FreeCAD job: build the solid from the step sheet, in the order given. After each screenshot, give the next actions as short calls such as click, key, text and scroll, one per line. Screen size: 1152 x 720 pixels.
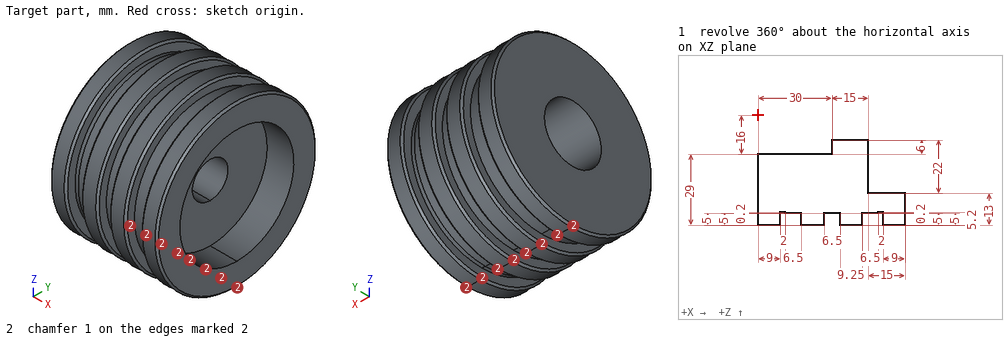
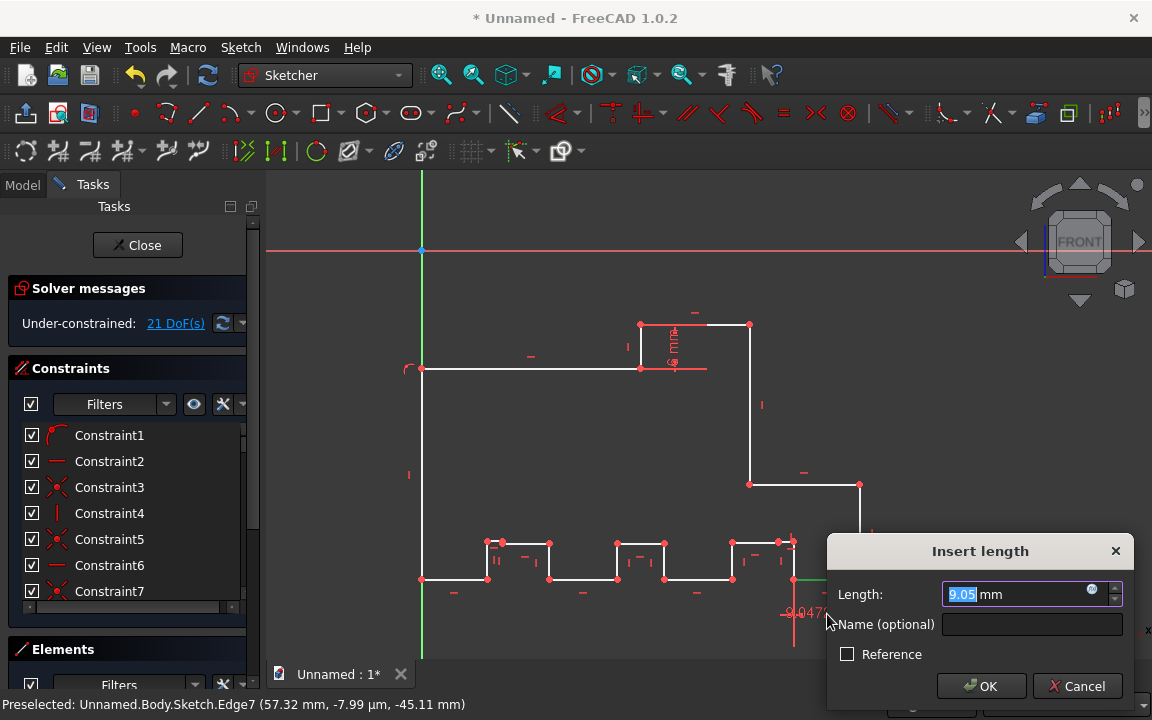
text(9)
key(Return)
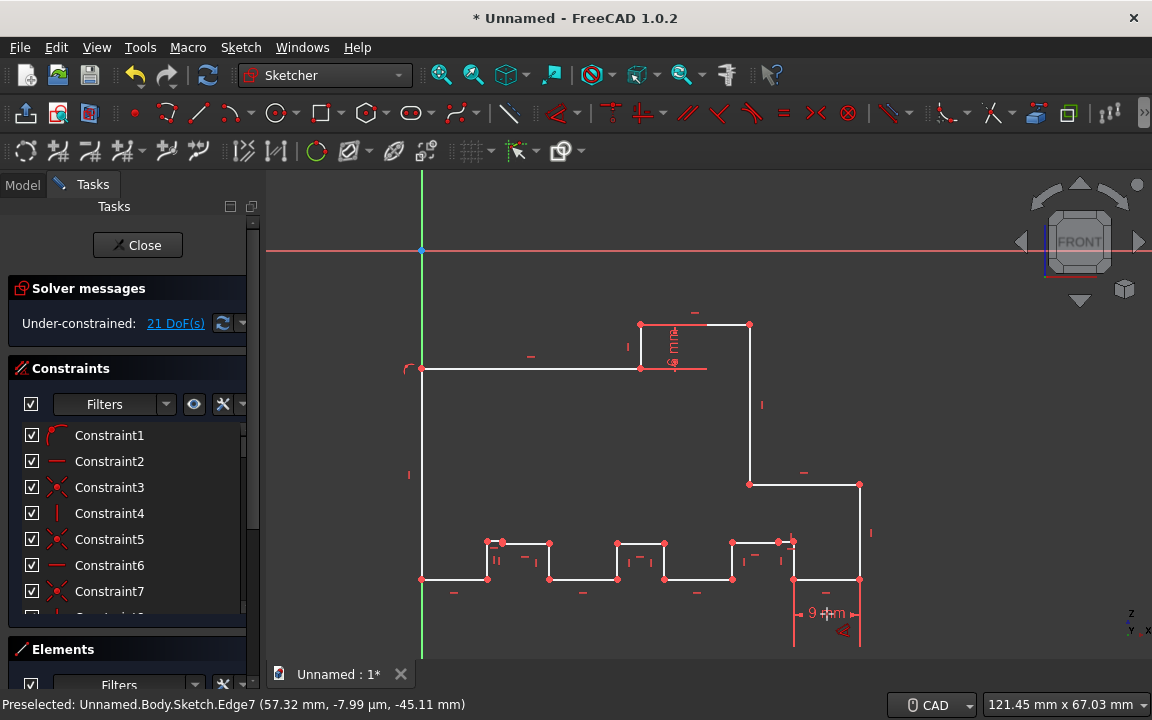
scroll(786, 542, up, 6)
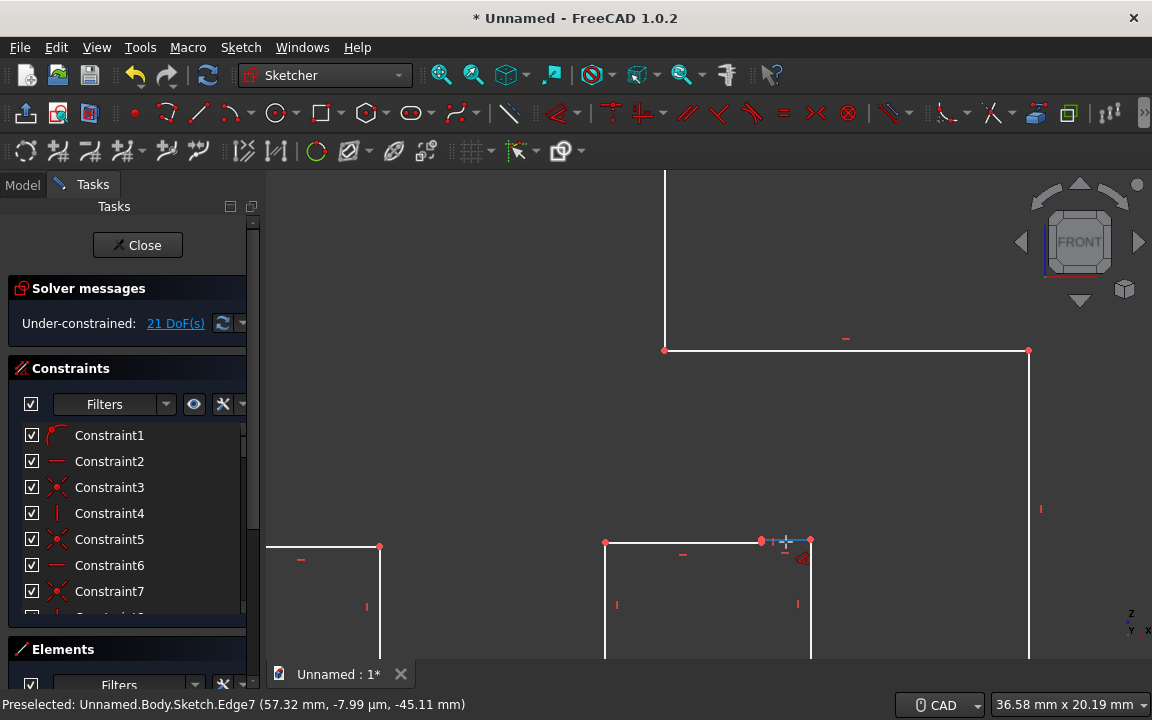
click(786, 540)
click(786, 574)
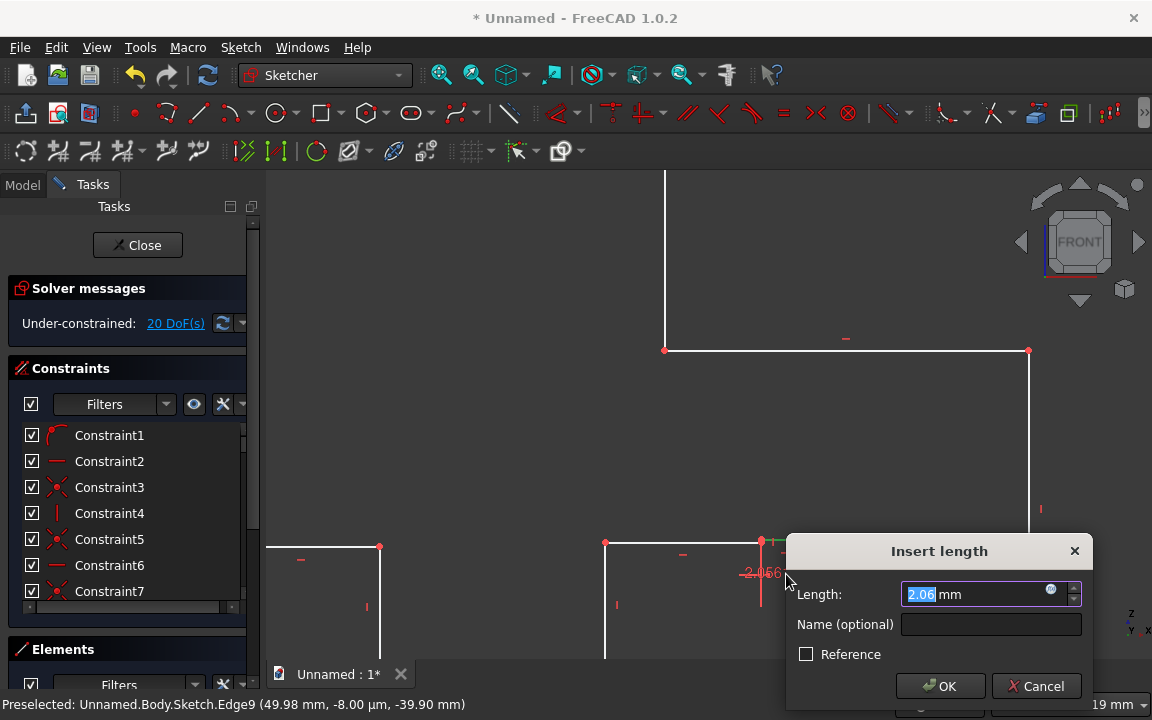
text(2)
key(Return)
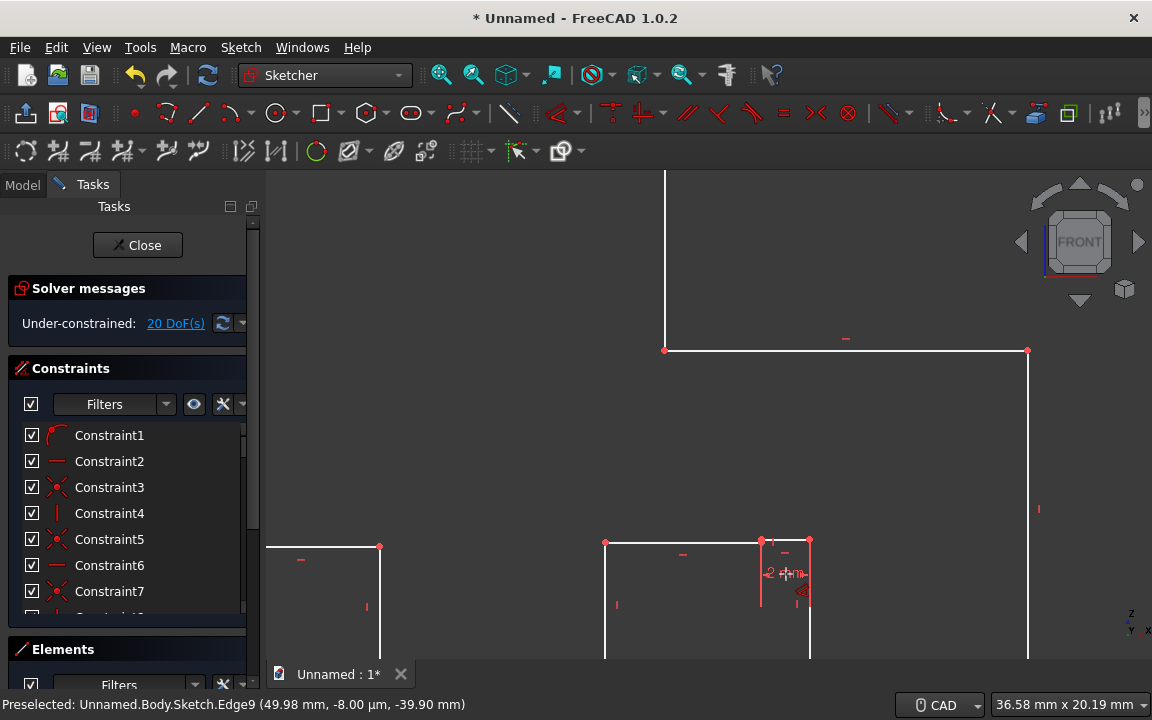
click(605, 580)
click(639, 587)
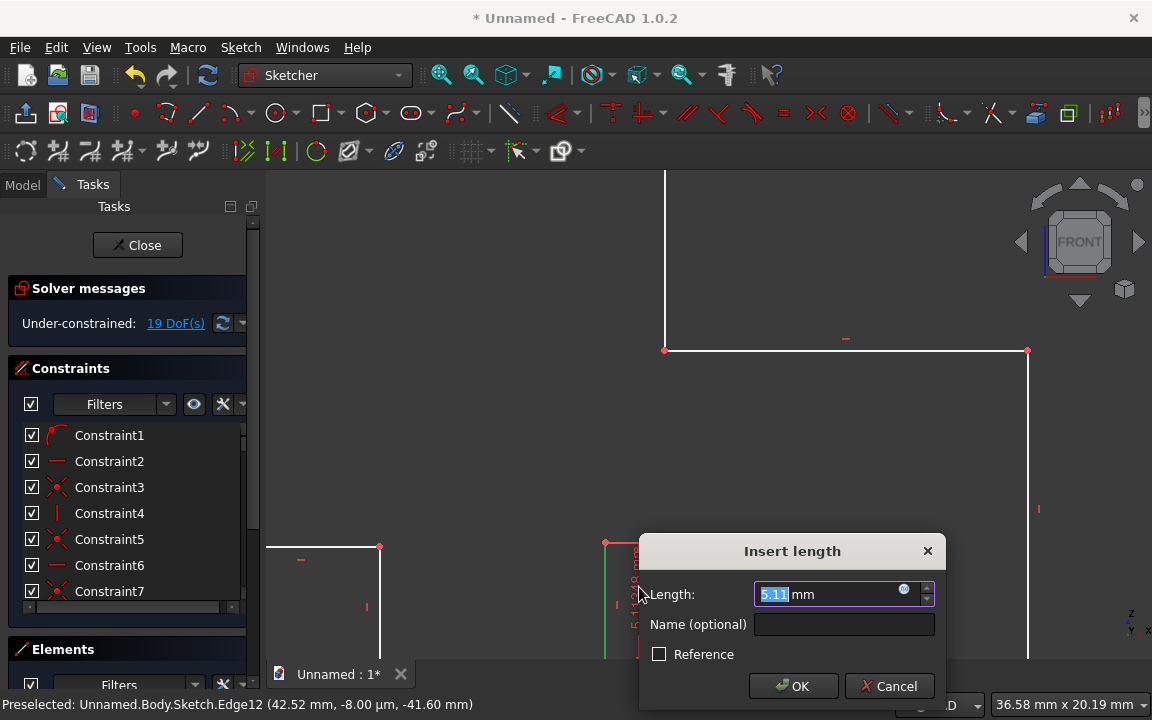
text(5)
key(Return)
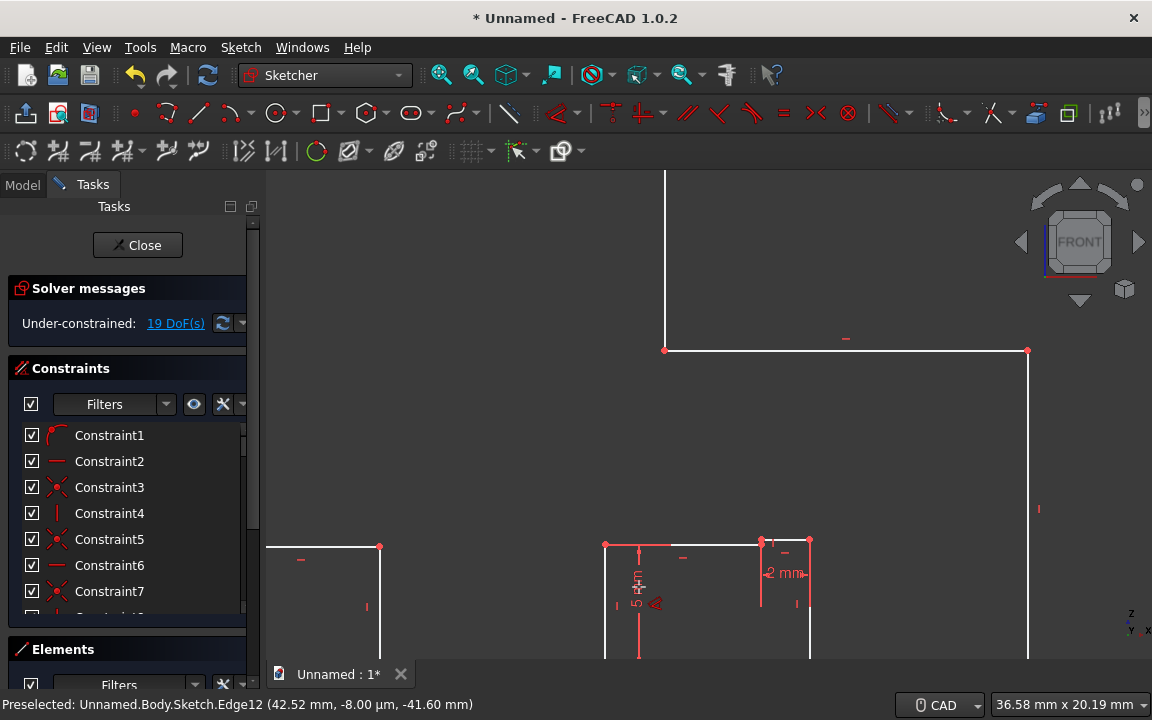
click(380, 630)
click(414, 589)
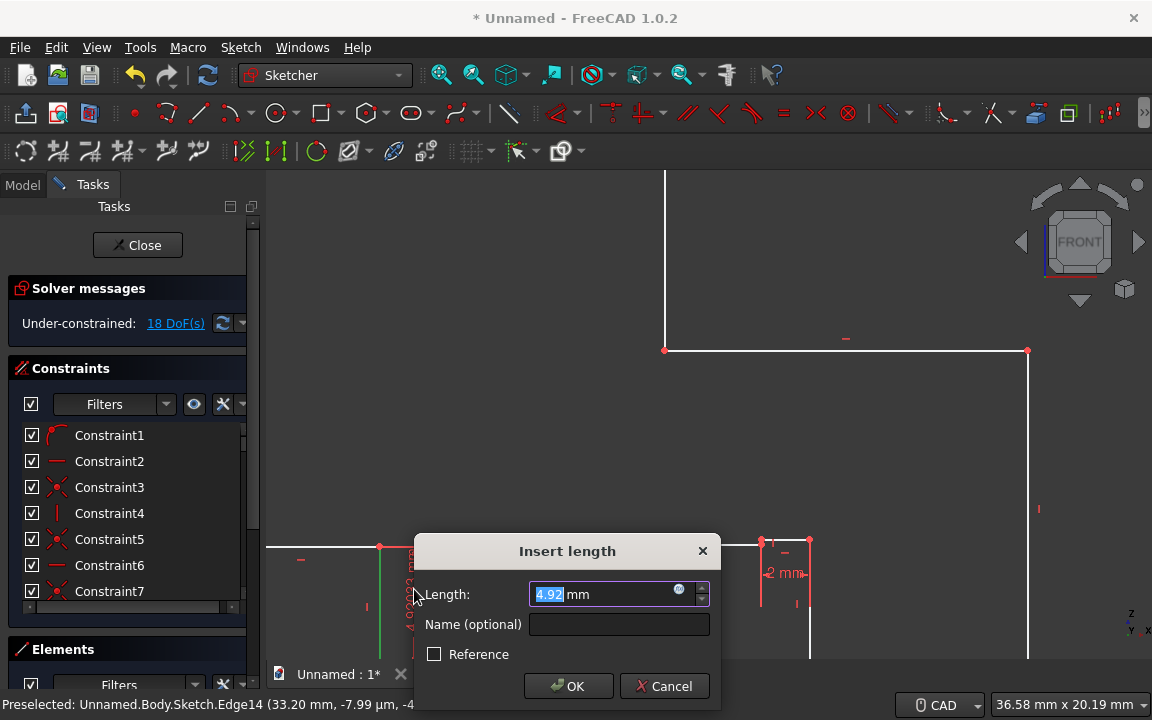
text(5)
key(Return)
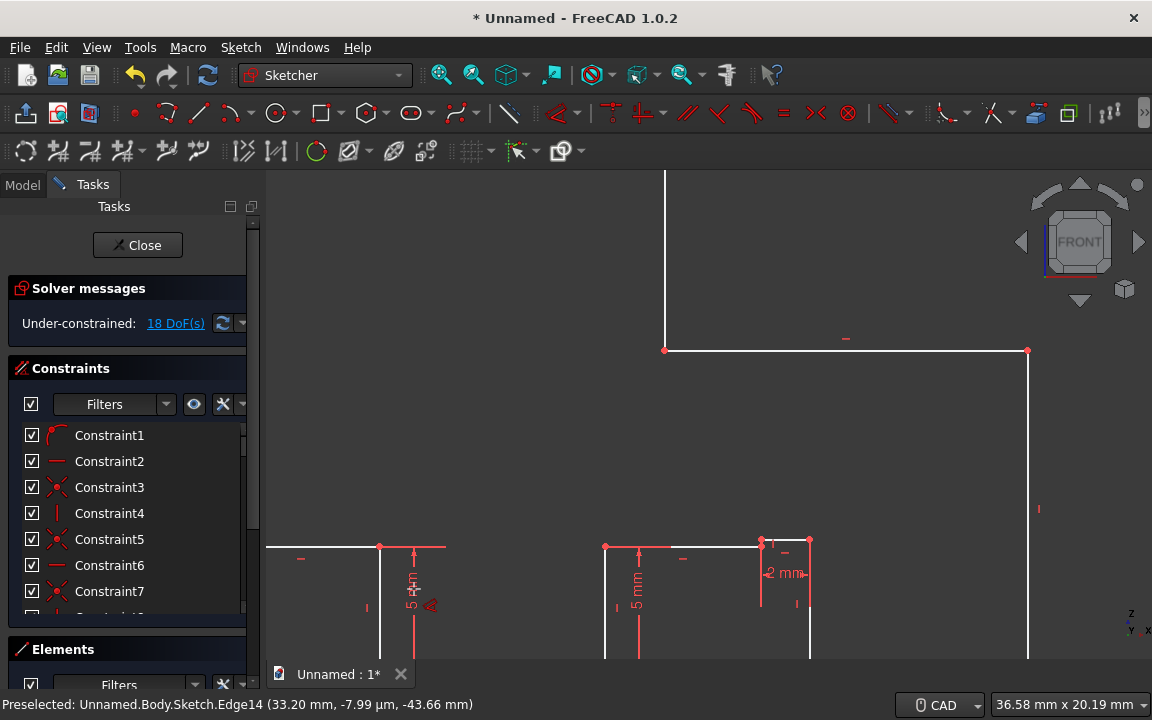
scroll(786, 542, down, 6)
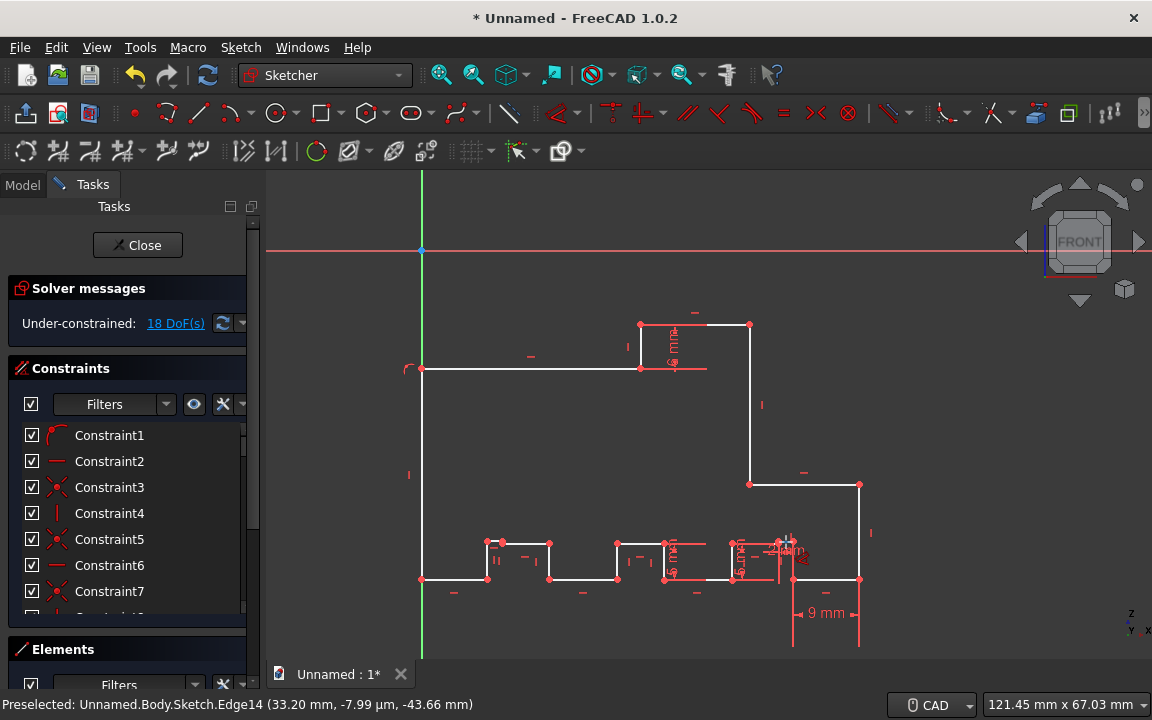
scroll(617, 555, up, 2)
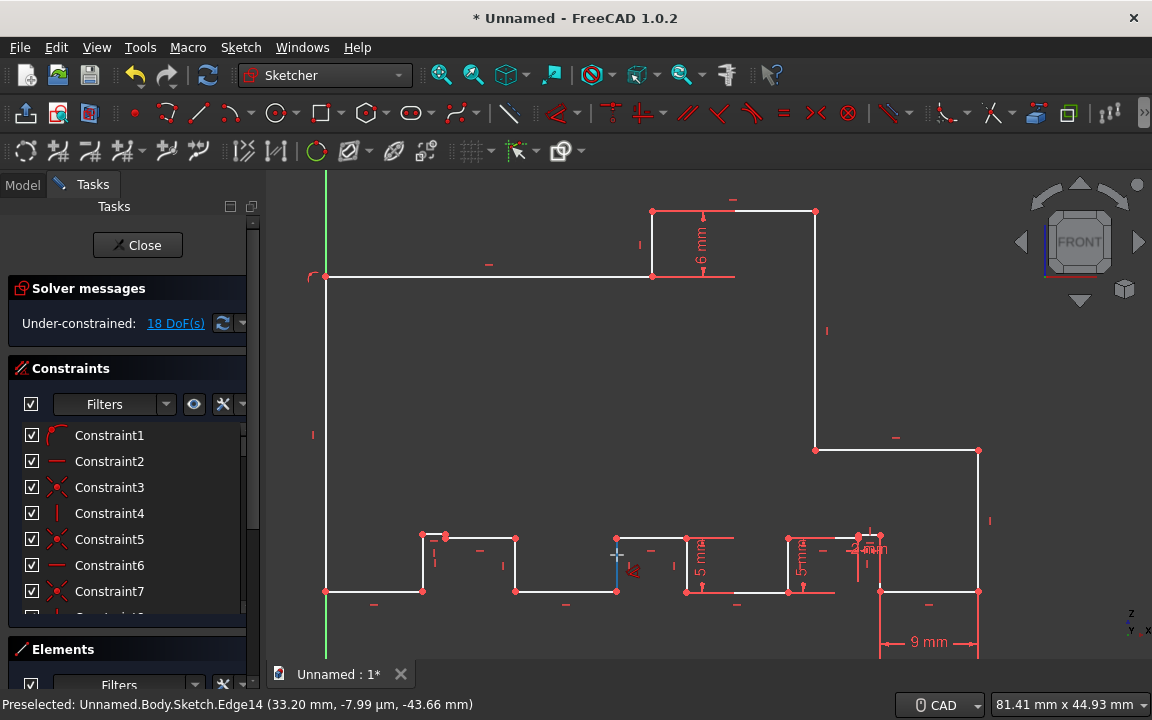
click(617, 554)
click(583, 565)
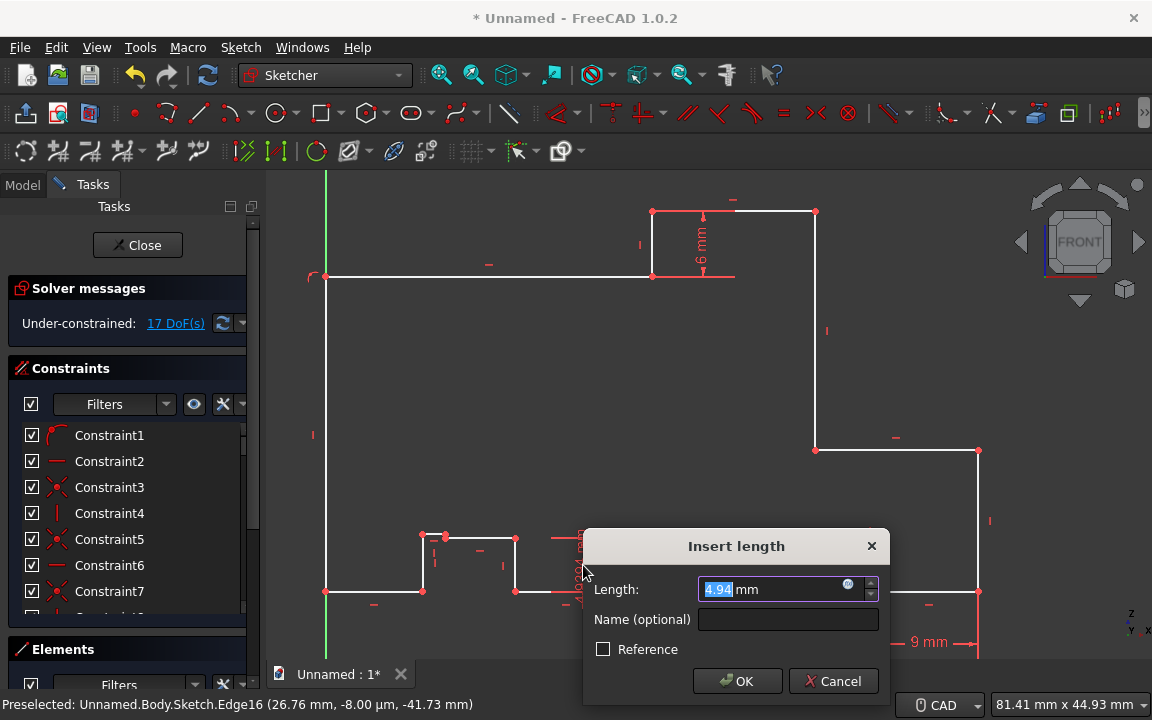
text(5)
key(Return)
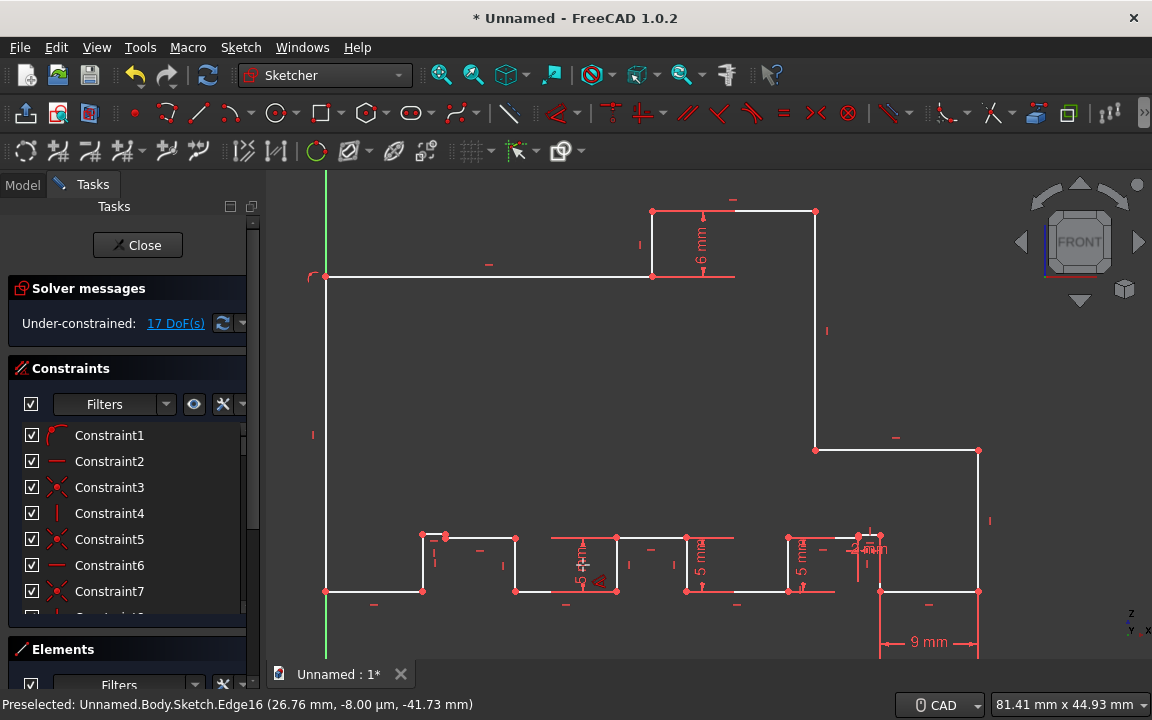
click(515, 576)
click(481, 565)